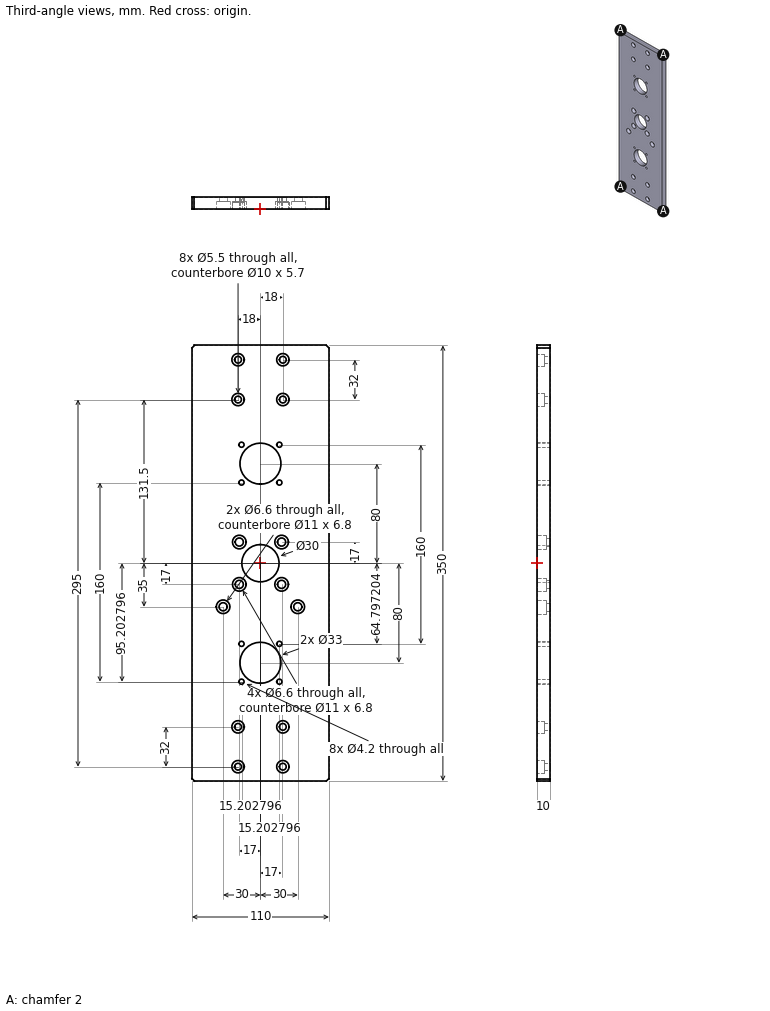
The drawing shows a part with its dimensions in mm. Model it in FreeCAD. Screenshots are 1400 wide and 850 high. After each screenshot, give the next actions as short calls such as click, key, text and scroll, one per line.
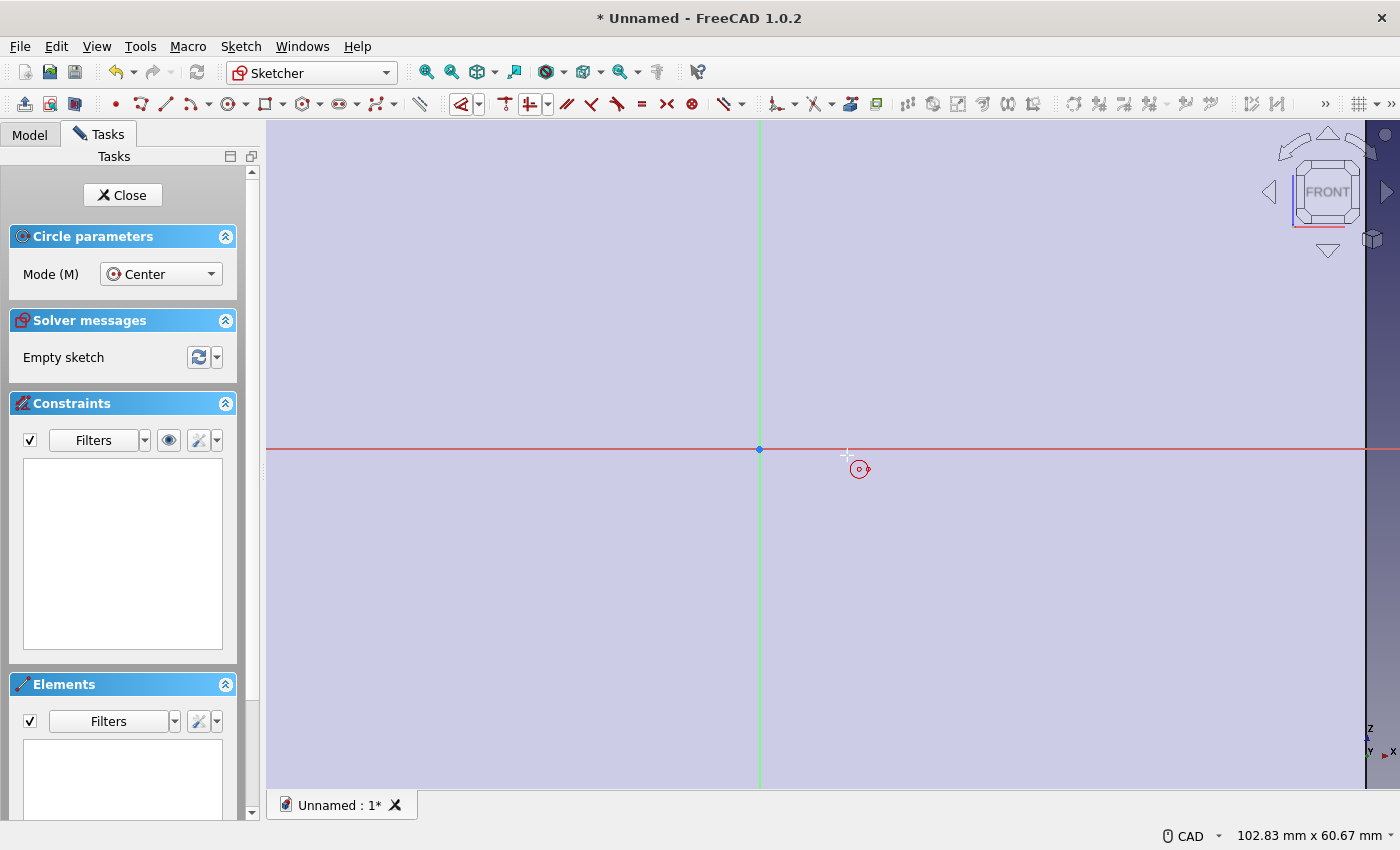
click(572, 637)
move(598, 611)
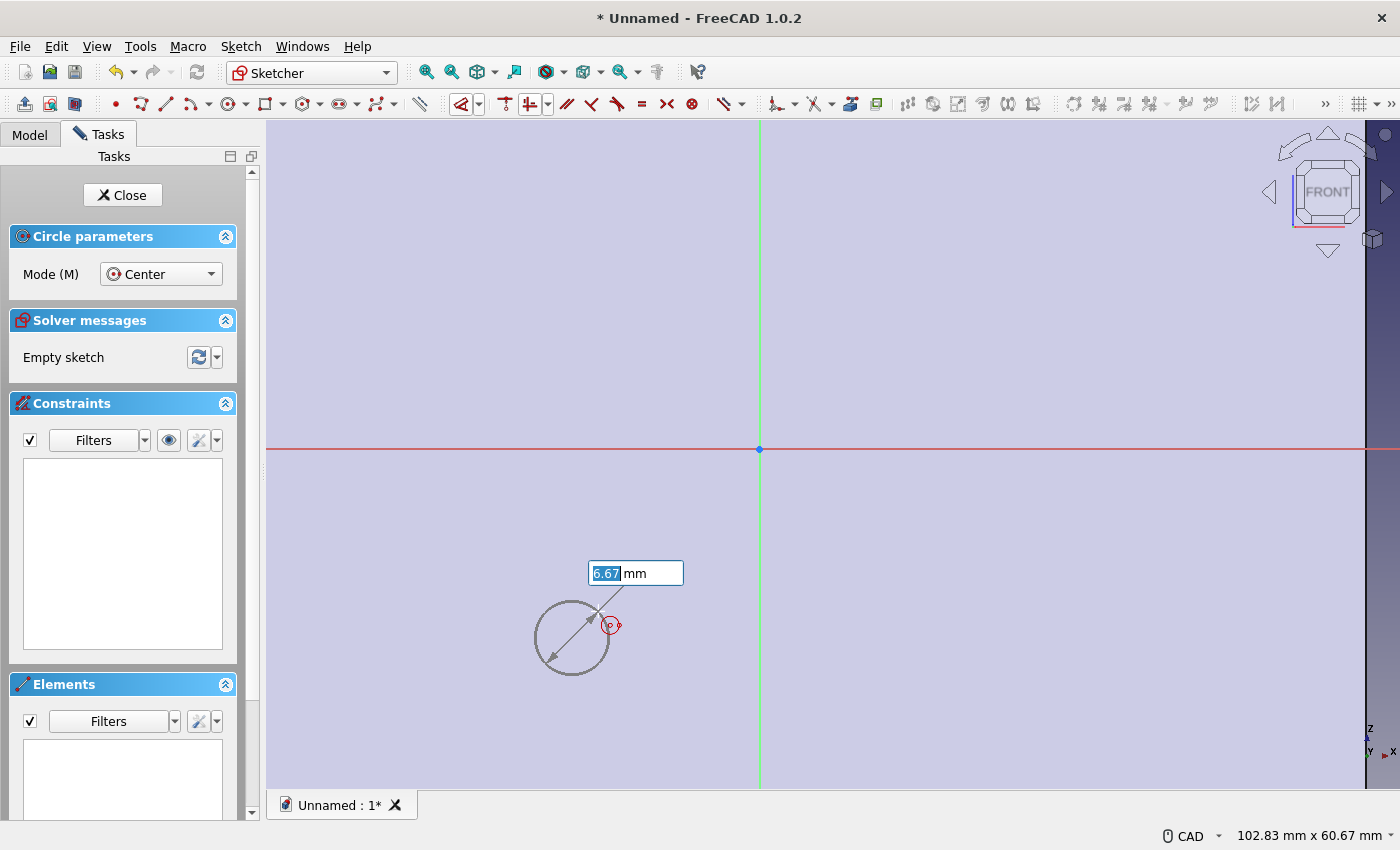
text(6.6)
key(Return)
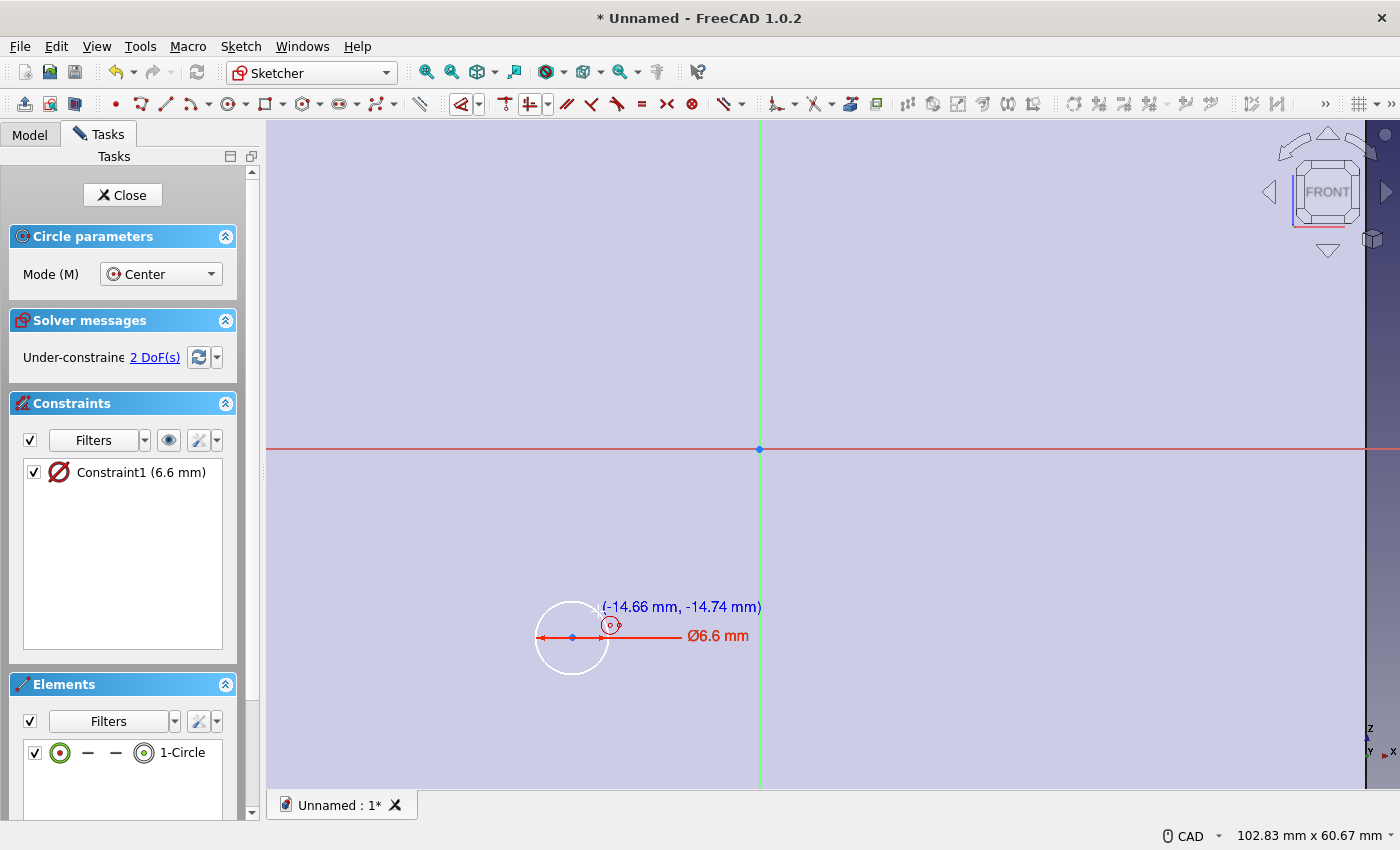
click(947, 637)
move(973, 611)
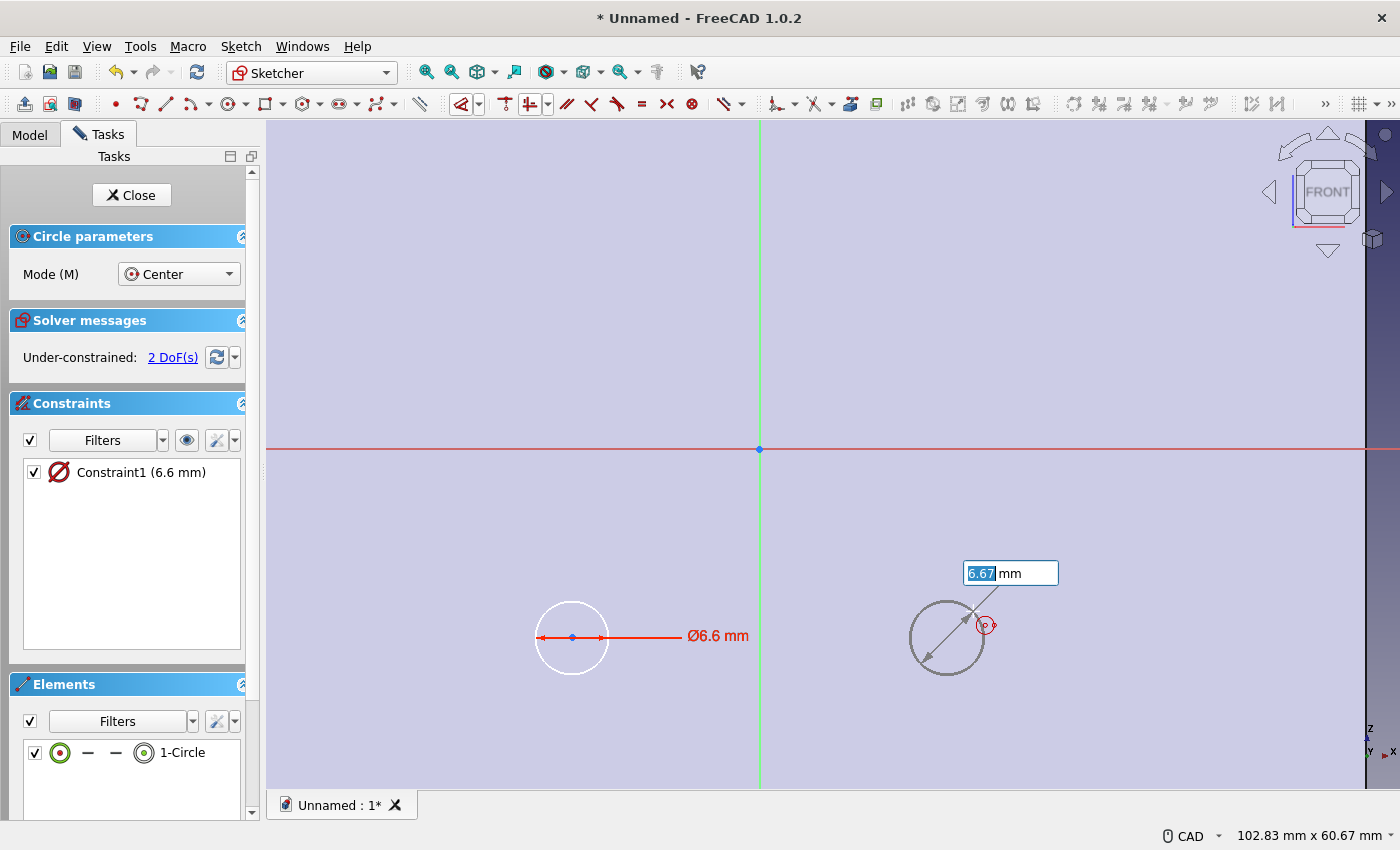
text(6.6)
key(Return)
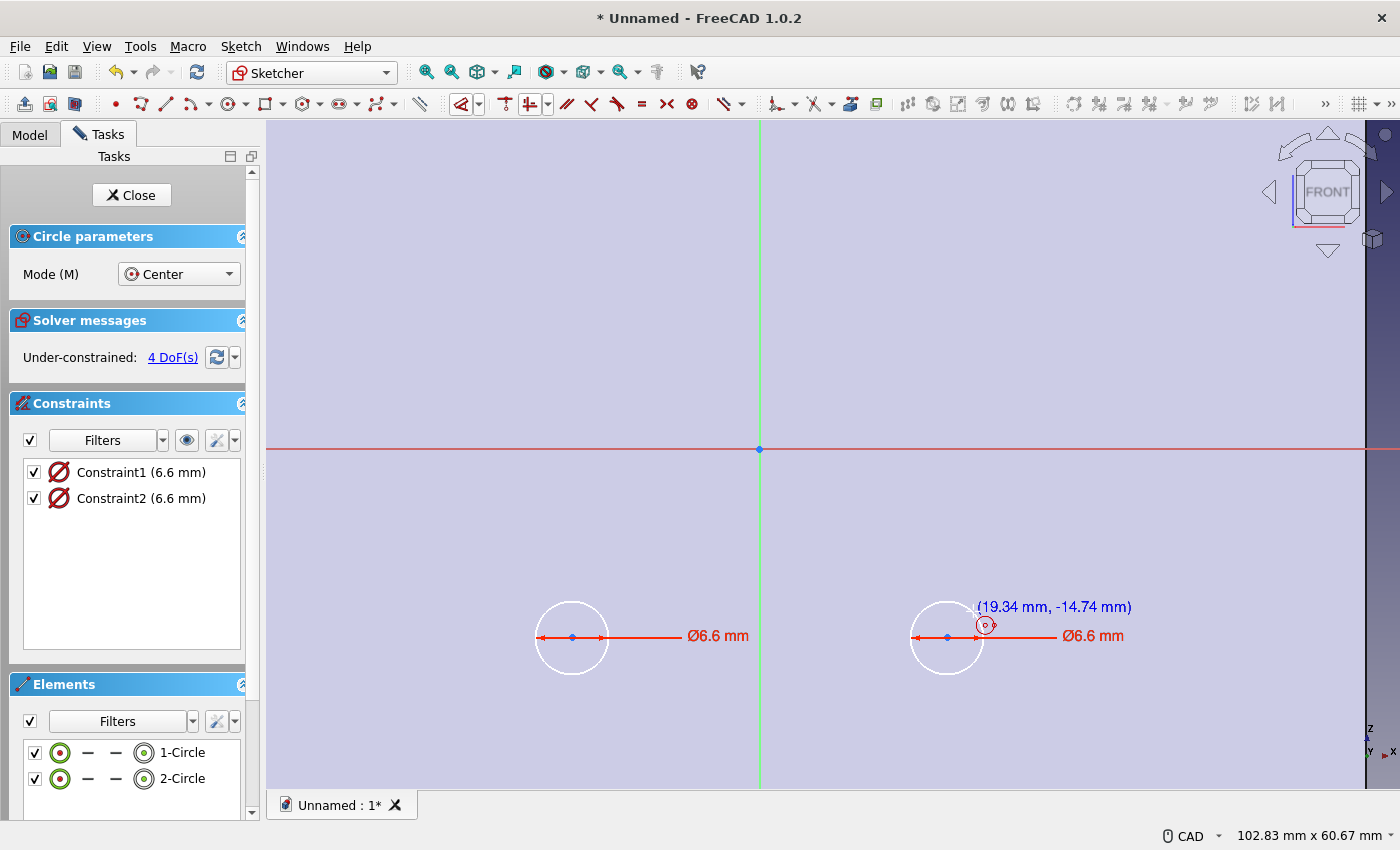
click(947, 262)
move(973, 236)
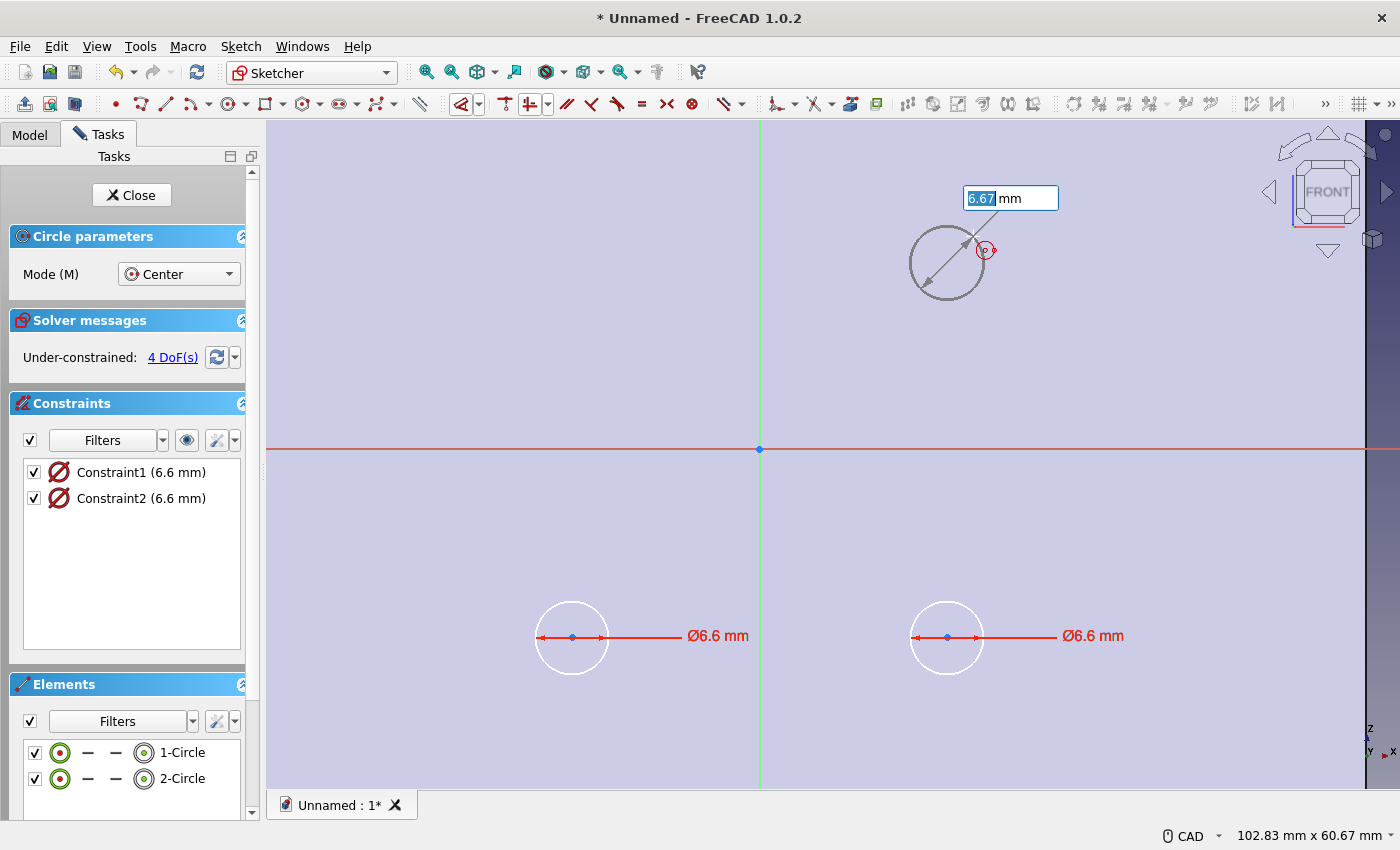
text(6.6)
key(Return)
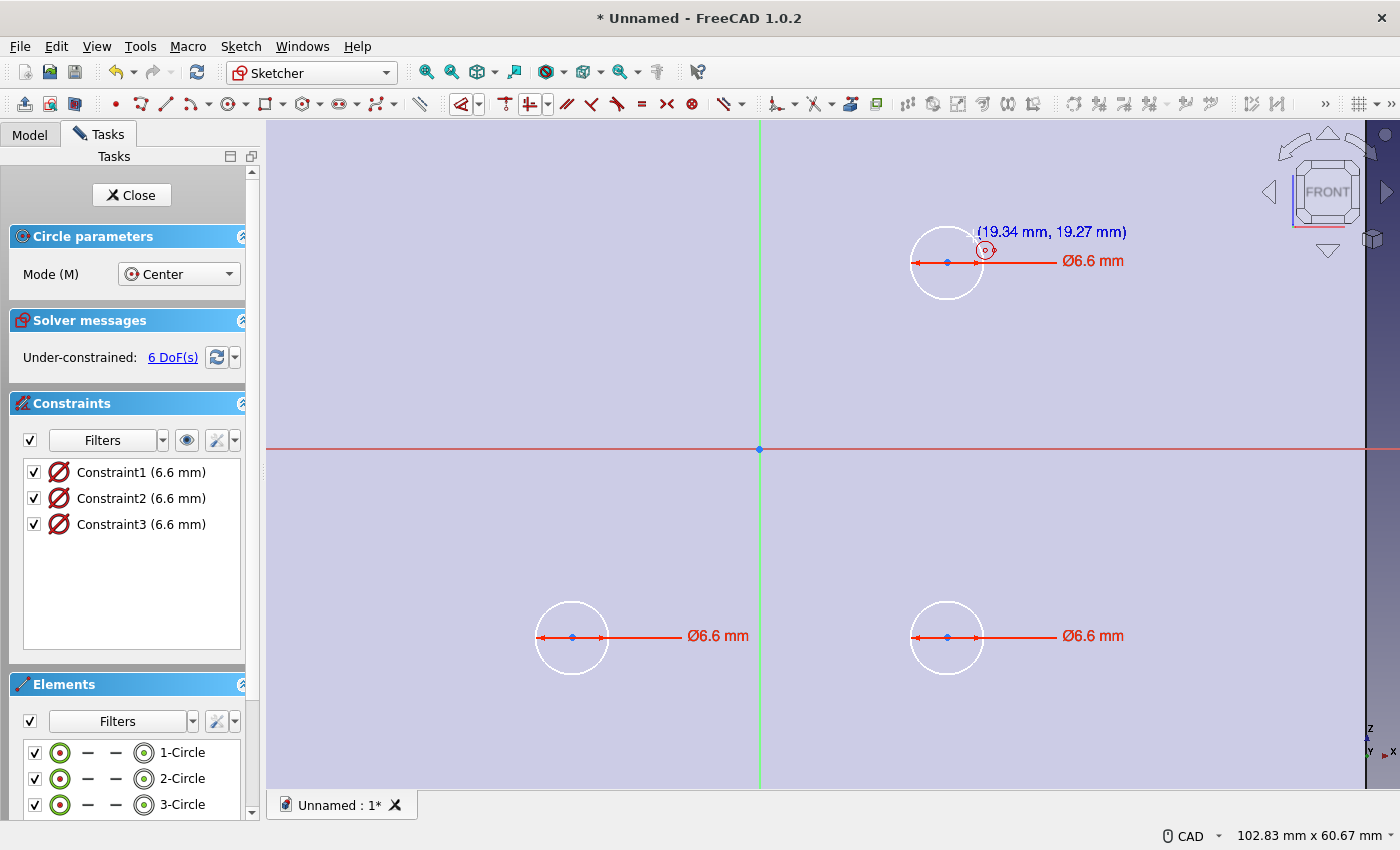
click(572, 262)
move(598, 236)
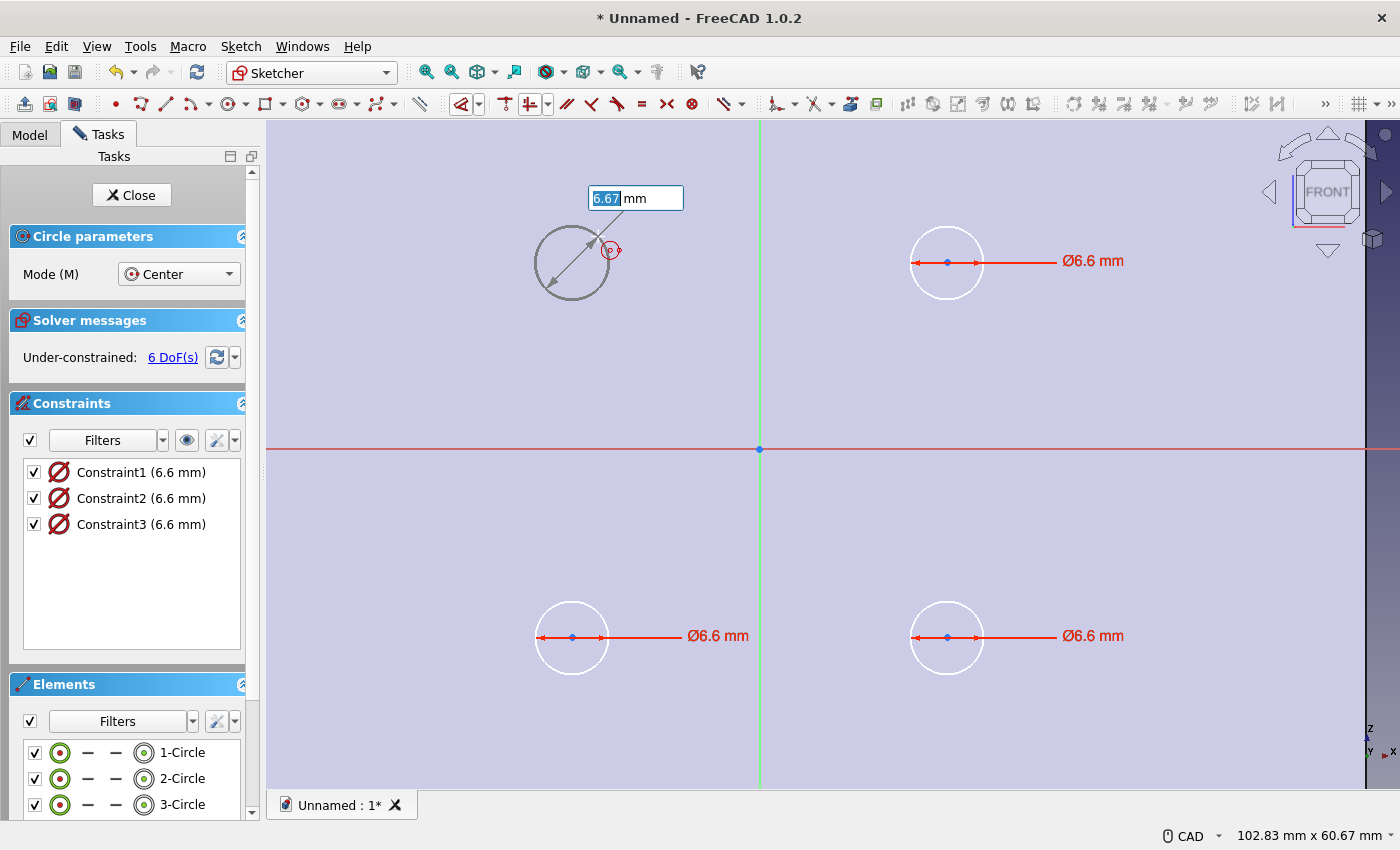
text(6.6)
key(Return)
key(Escape)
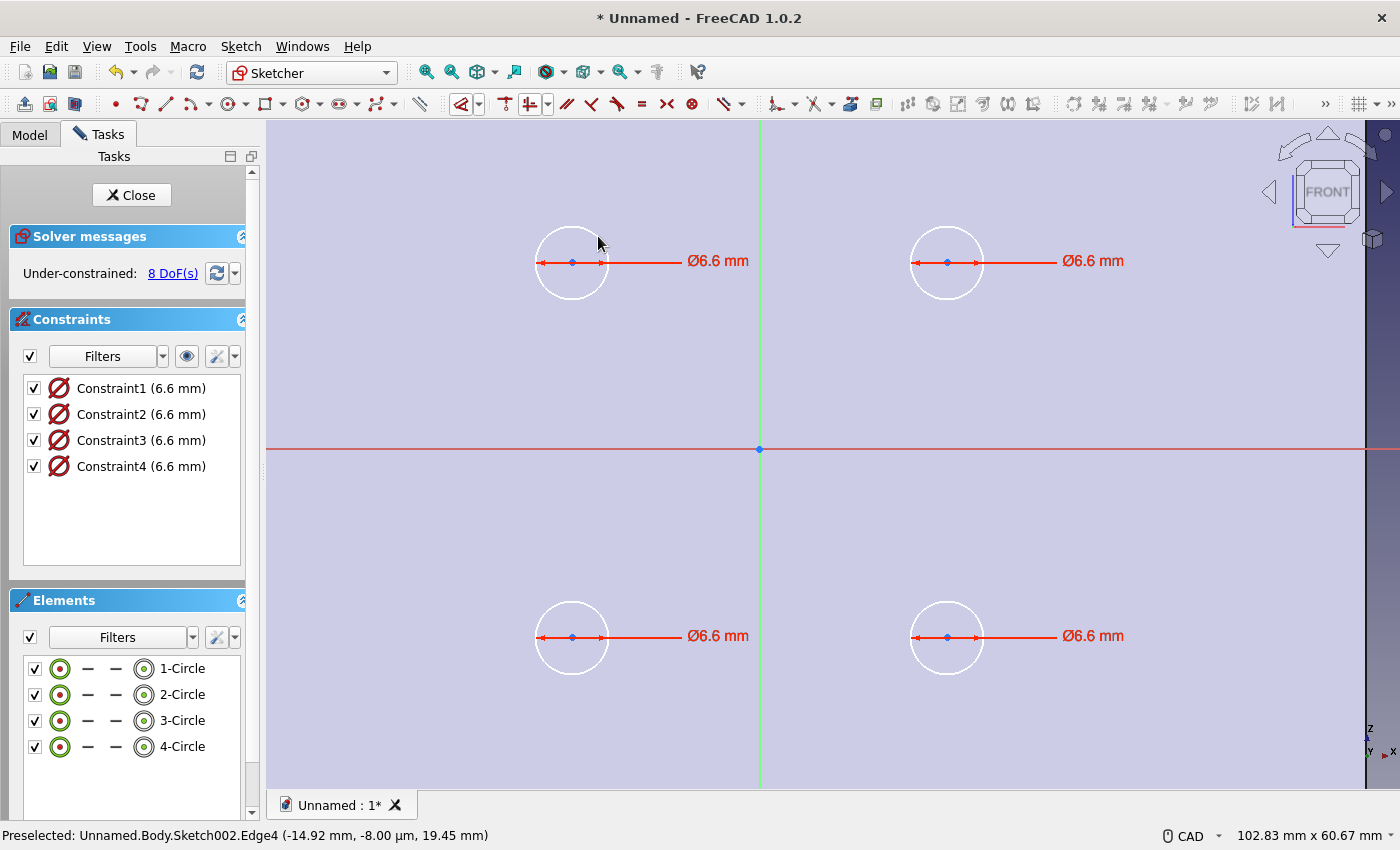
click(572, 638)